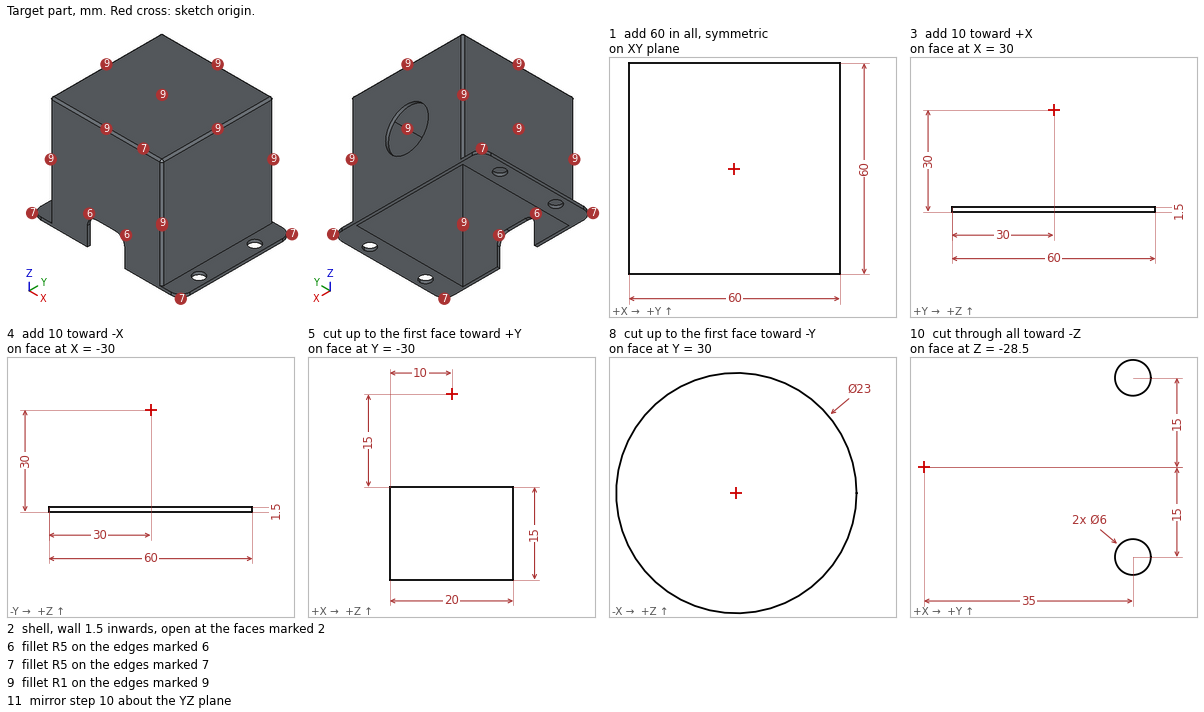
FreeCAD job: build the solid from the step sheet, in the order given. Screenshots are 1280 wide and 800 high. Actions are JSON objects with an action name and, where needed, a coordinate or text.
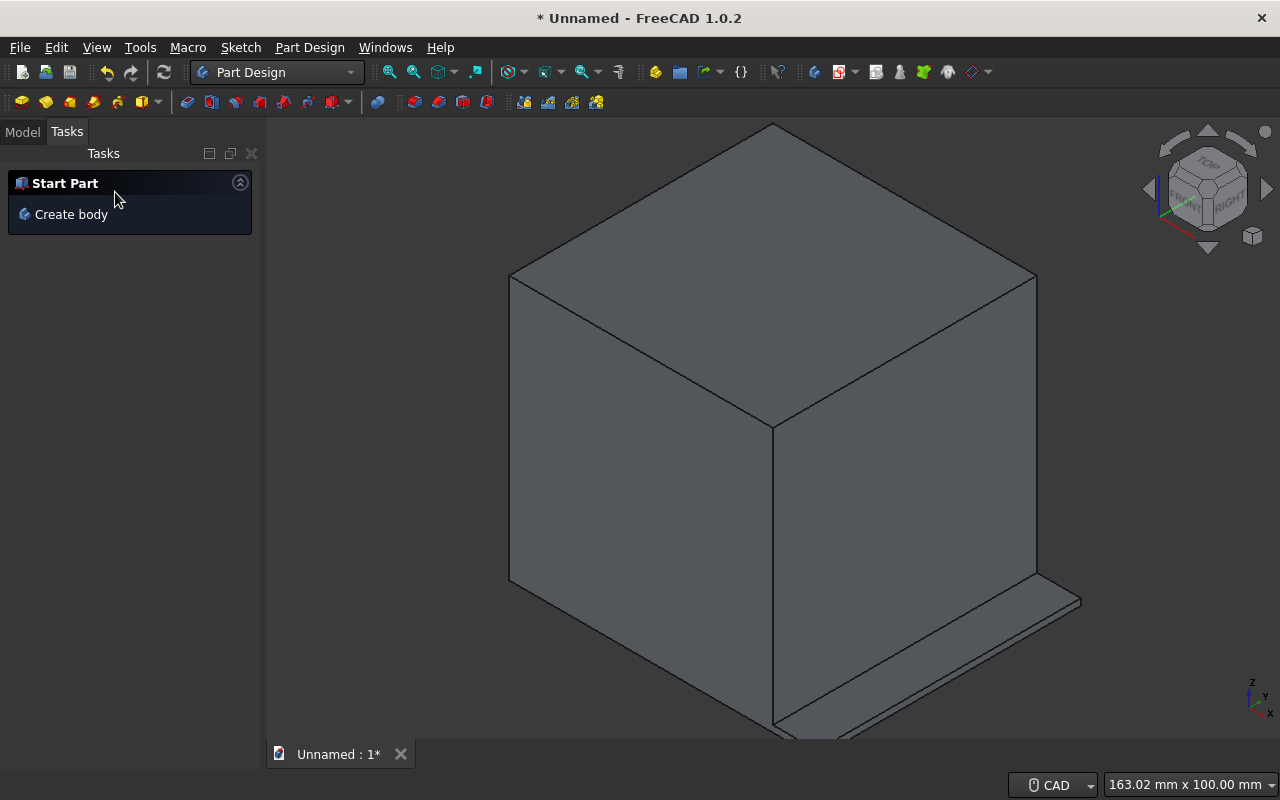
{"action": "left_click", "coordinate": [390, 72]}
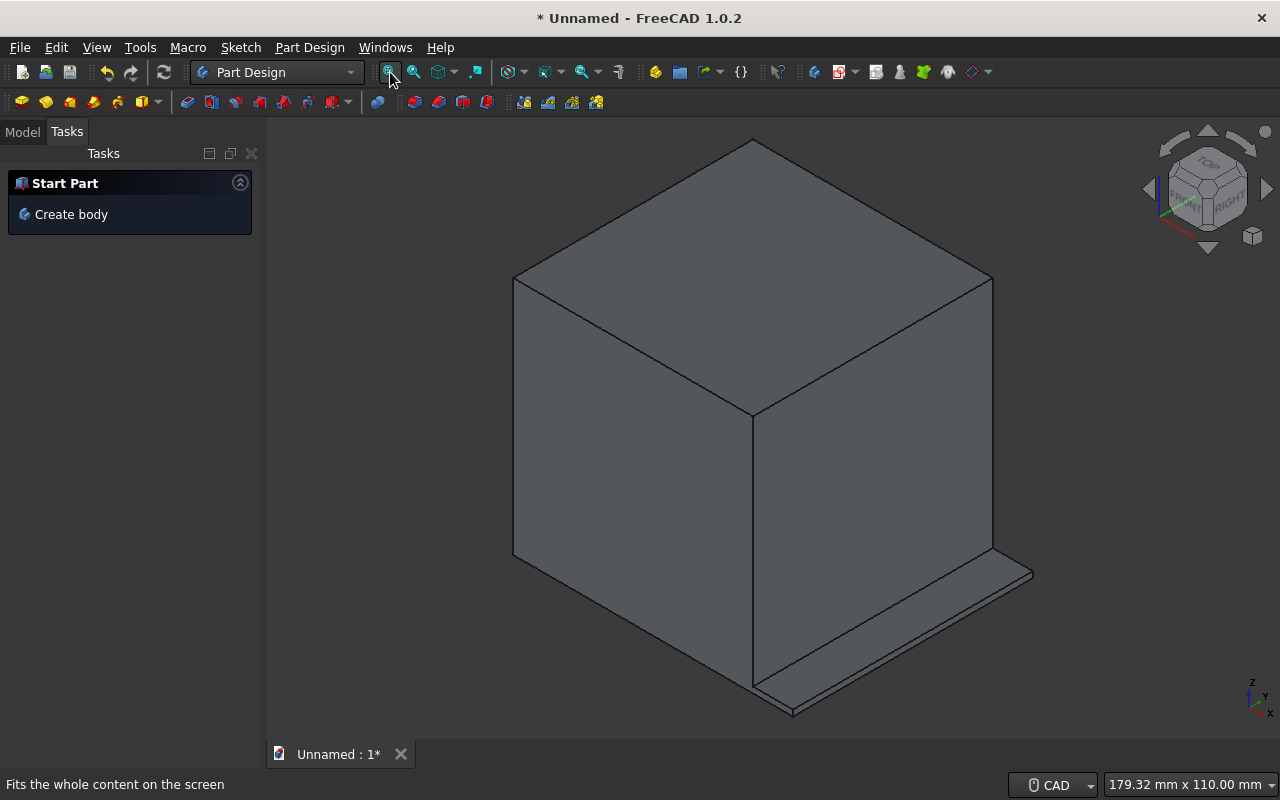
{"action": "key", "text": "6"}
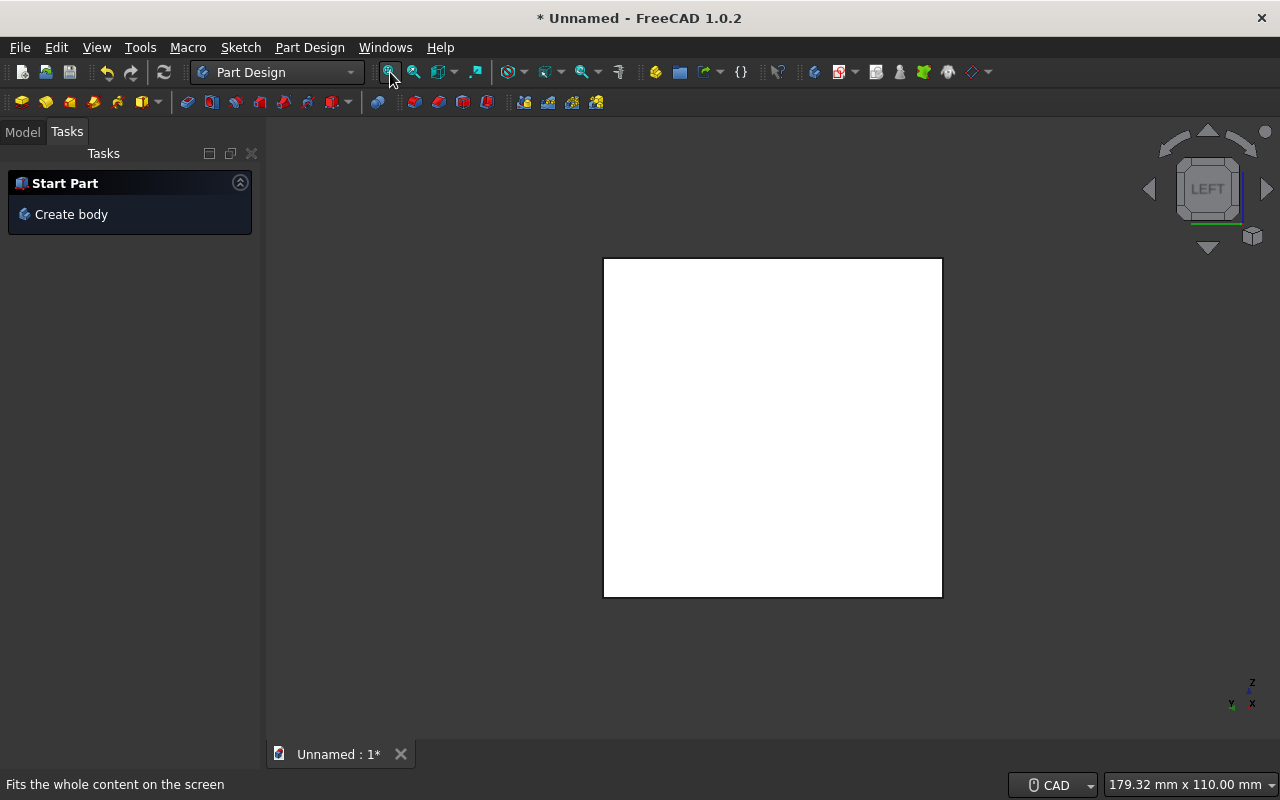
{"action": "left_click", "coordinate": [773, 427]}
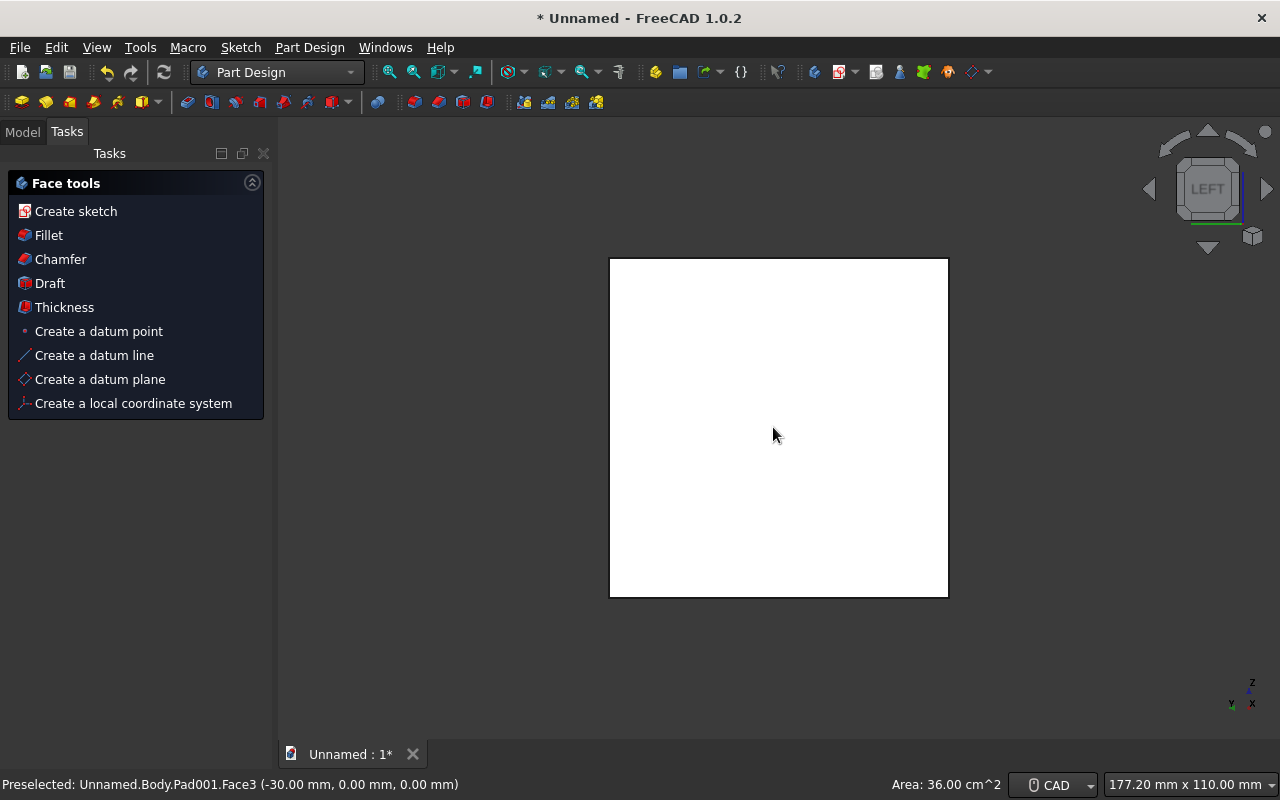
{"action": "left_click", "coordinate": [840, 72]}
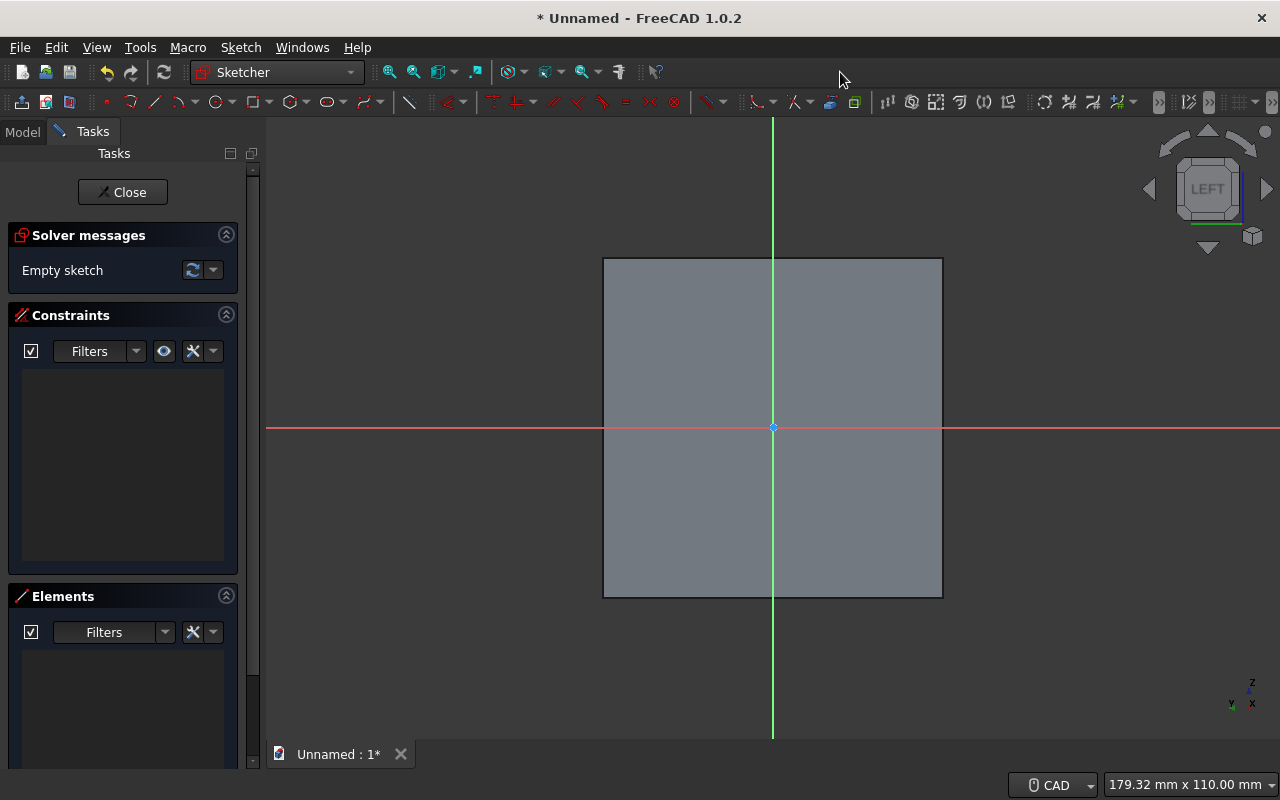
{"action": "scroll", "coordinate": [856, 616], "scroll_direction": "up", "scroll_amount": 3}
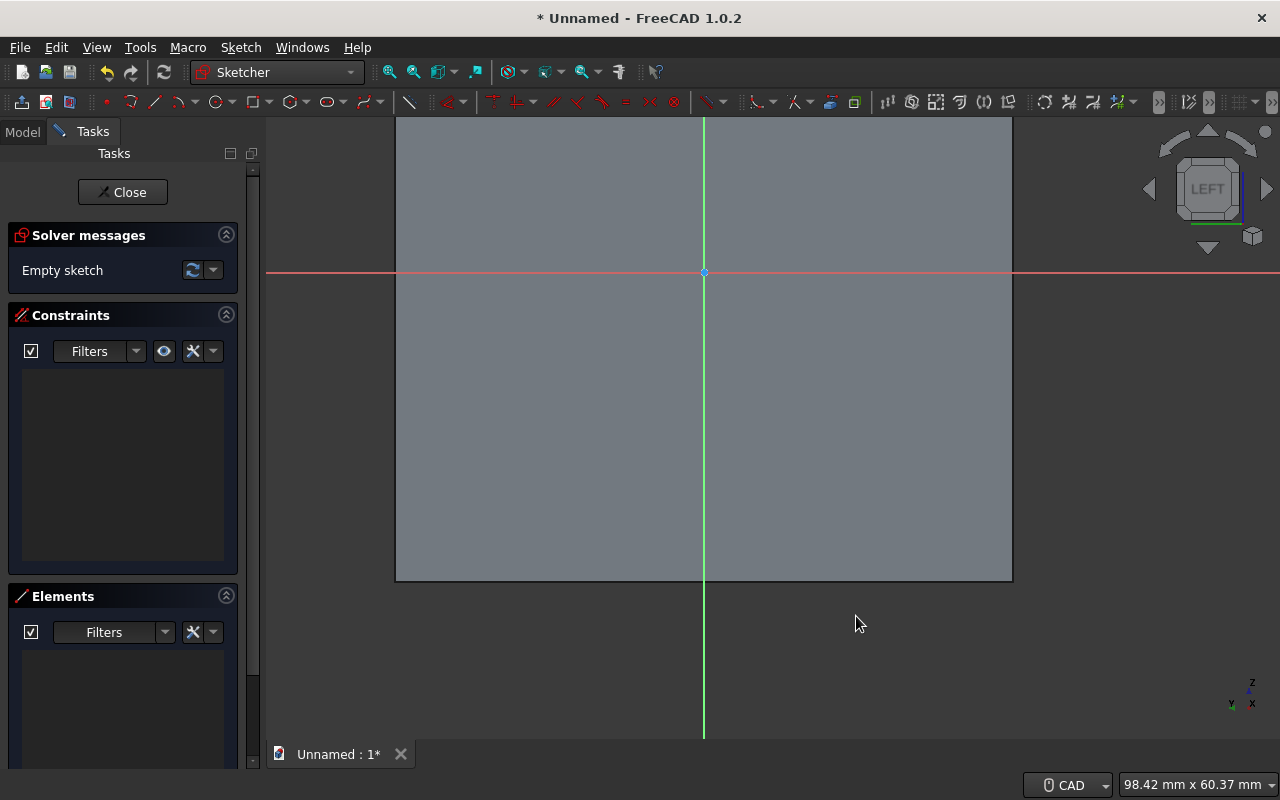
{"action": "key", "text": "g r"}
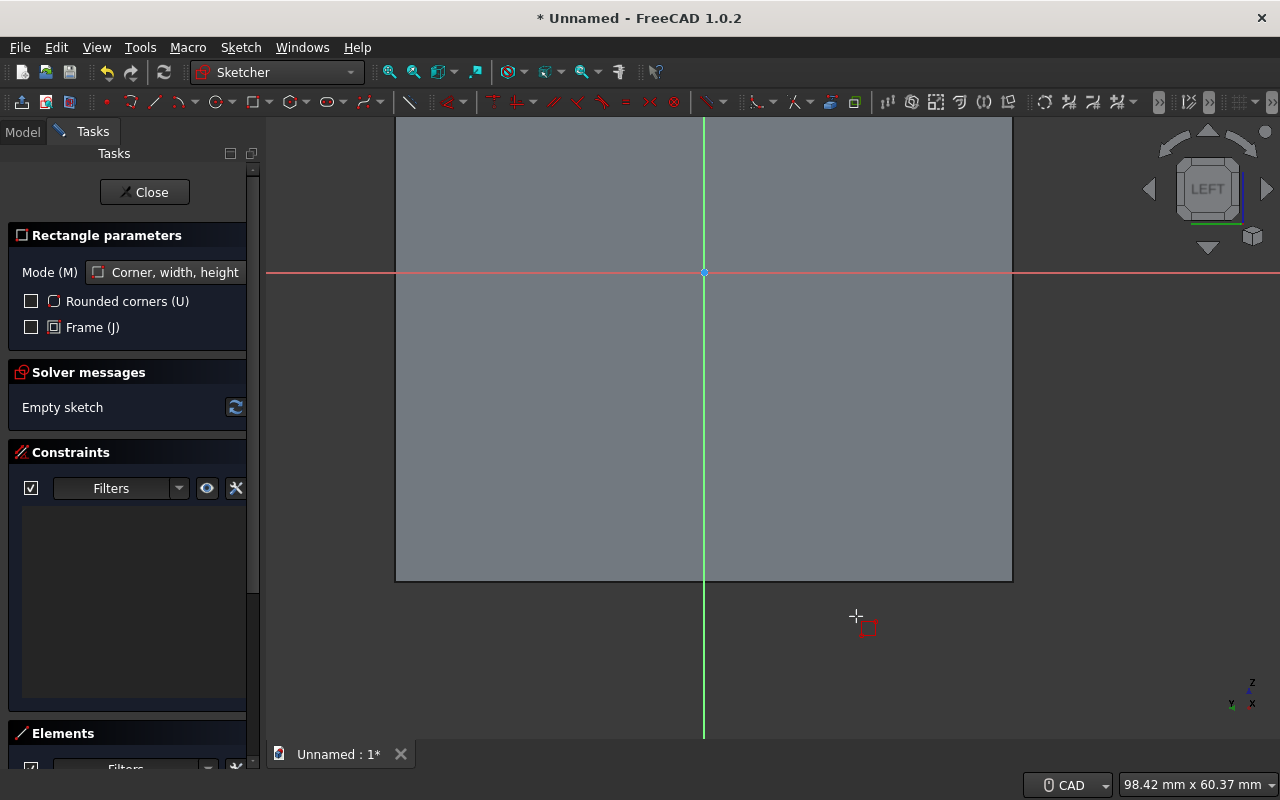
{"action": "left_click", "coordinate": [395, 566]}
{"action": "mouse_move", "coordinate": [1013, 582]}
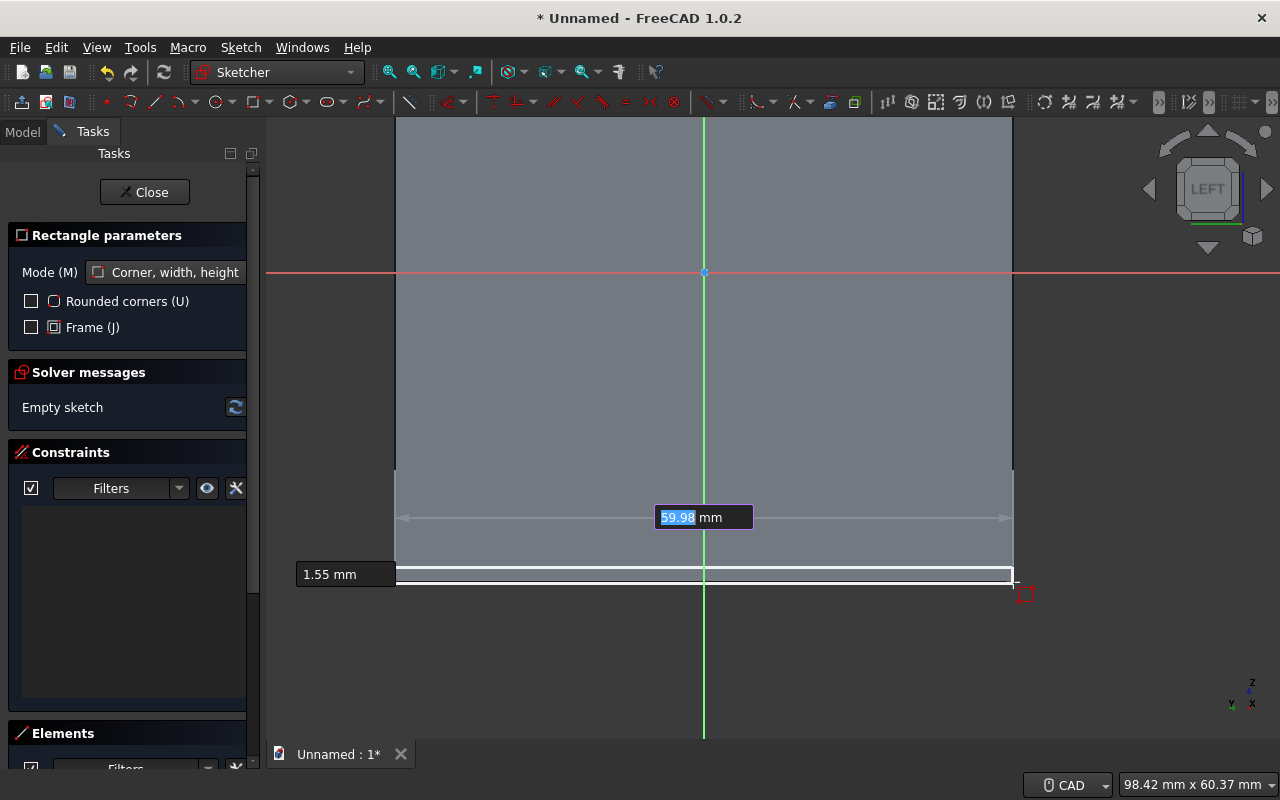
{"action": "type", "text": "60"}
{"action": "key", "text": "Tab"}
{"action": "type", "text": "1.5"}
{"action": "key", "text": "Return"}
{"action": "key", "text": "Escape"}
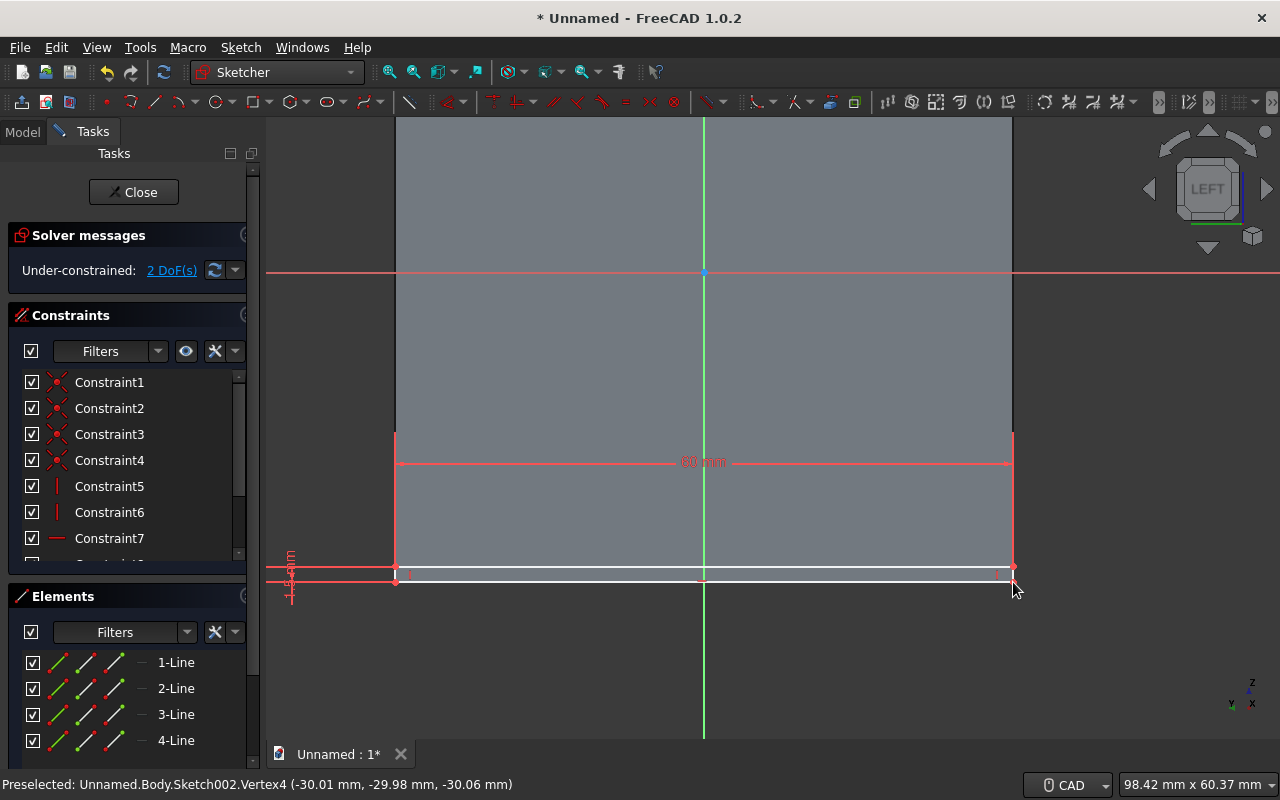
{"action": "left_click", "coordinate": [395, 567]}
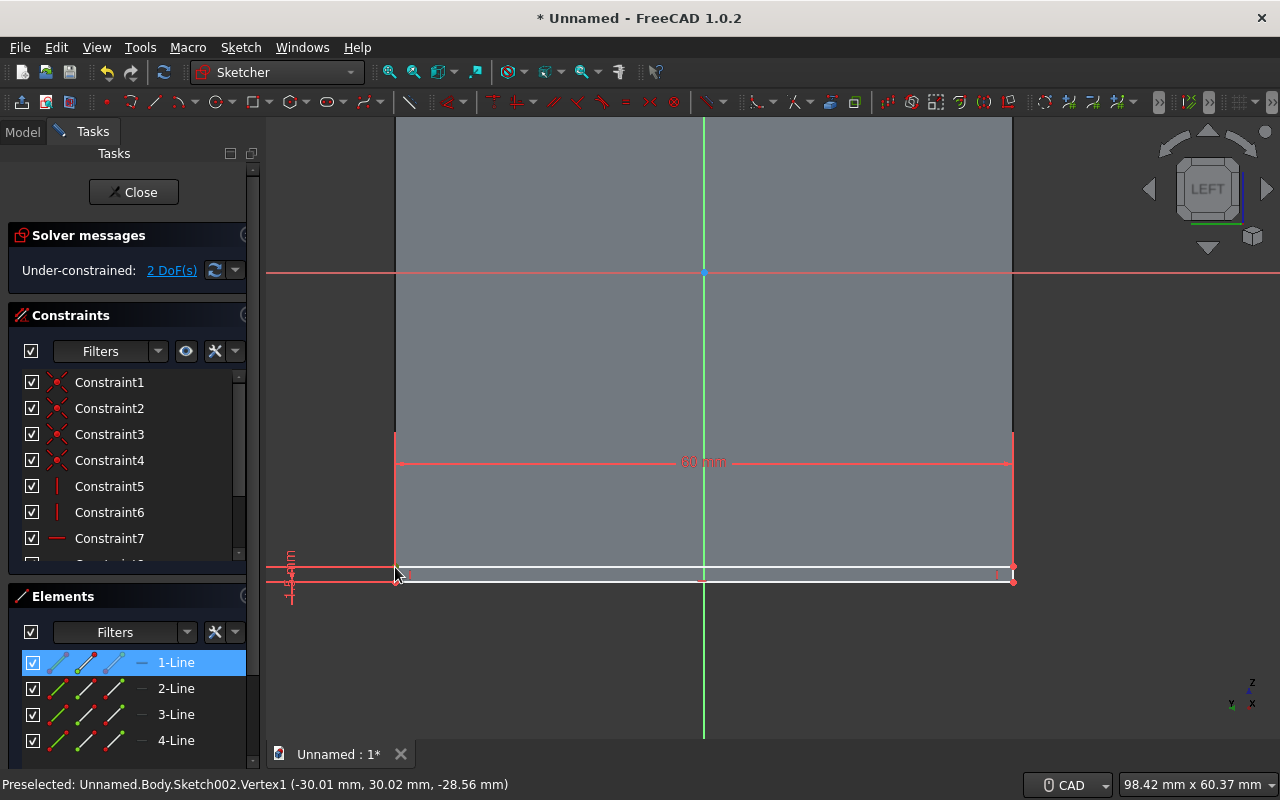
{"action": "key", "text": "l"}